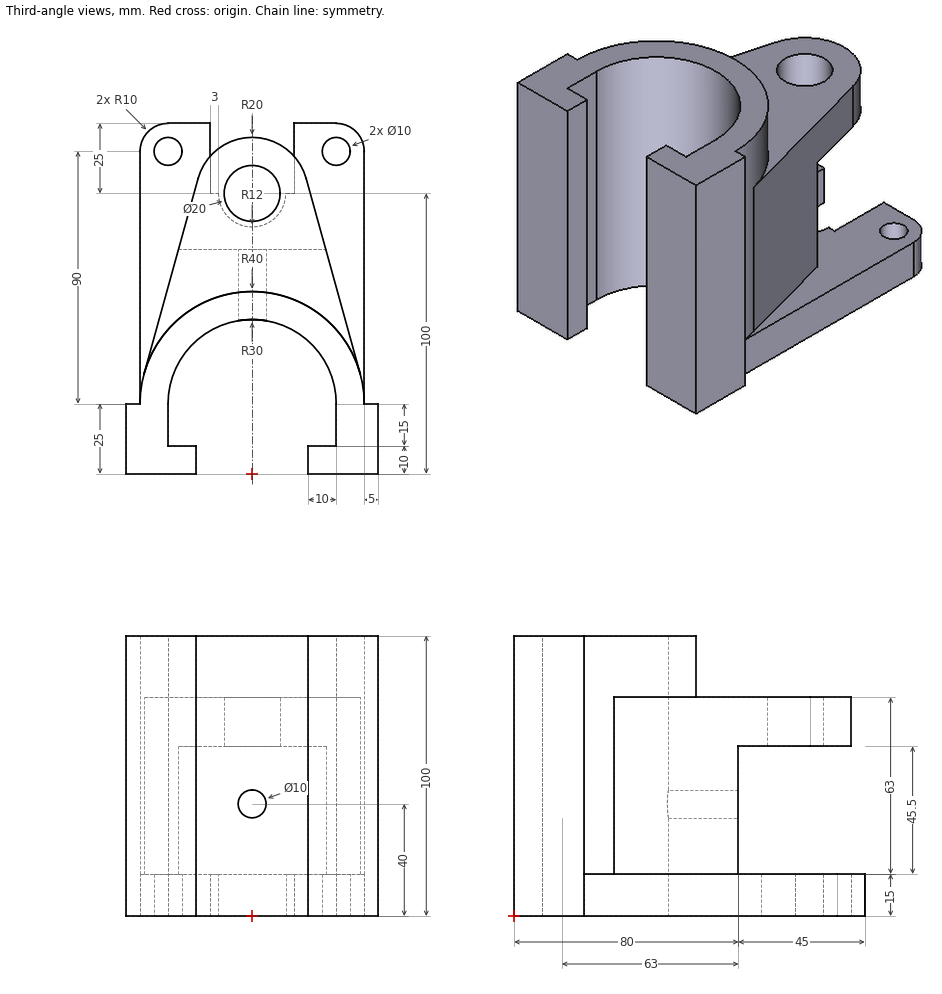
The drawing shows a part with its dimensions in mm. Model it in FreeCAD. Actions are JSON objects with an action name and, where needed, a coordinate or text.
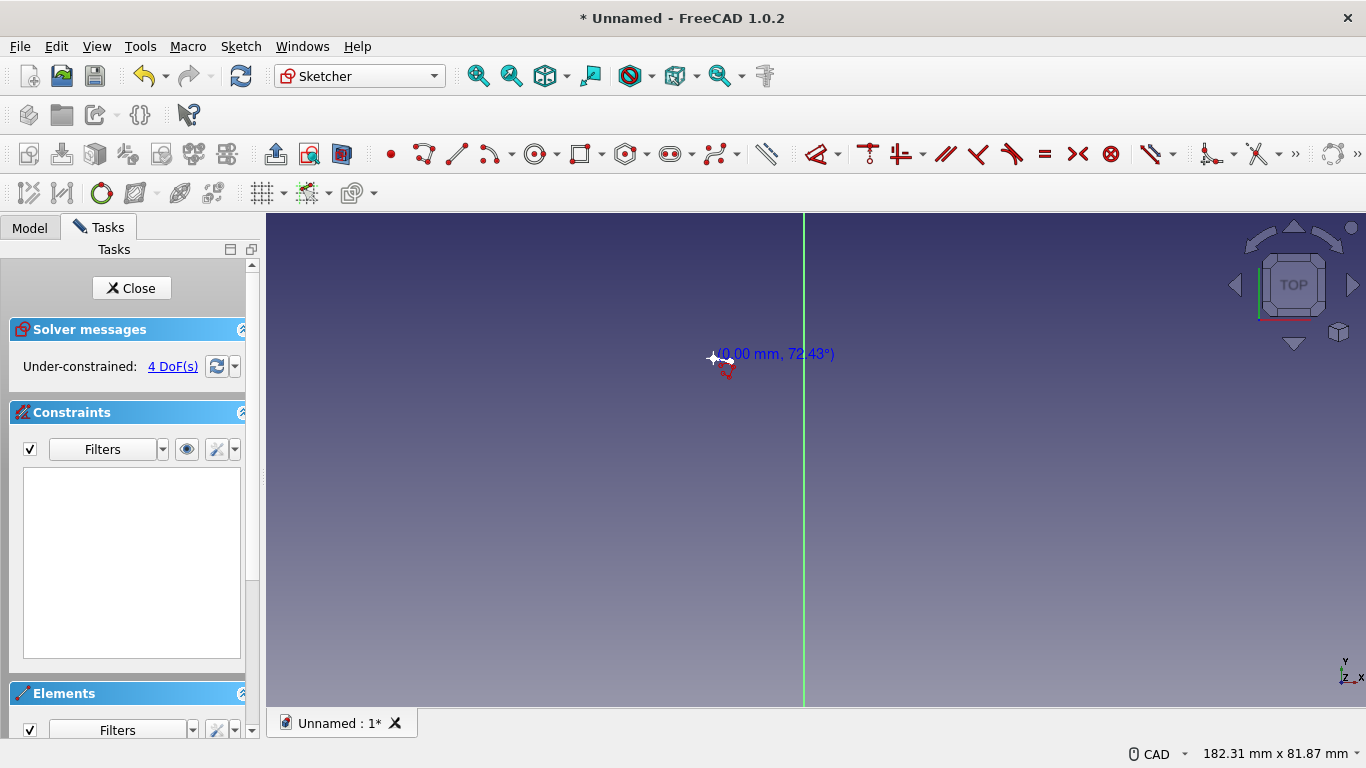
{"action": "scroll", "coordinate": [702, 358], "scroll_direction": "down", "scroll_amount": 4}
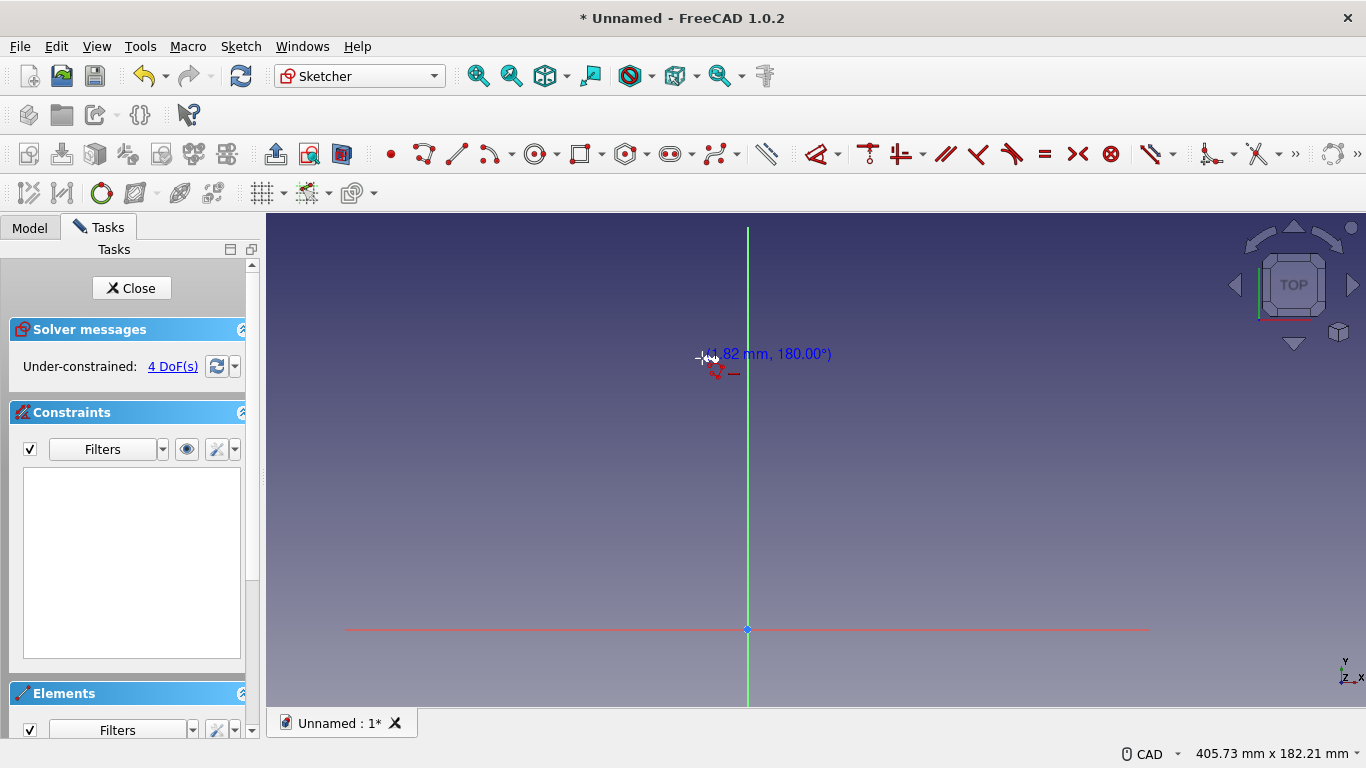
{"action": "left_click", "coordinate": [707, 291]}
{"action": "left_click", "coordinate": [667, 291]}
{"action": "right_click", "coordinate": [667, 291]}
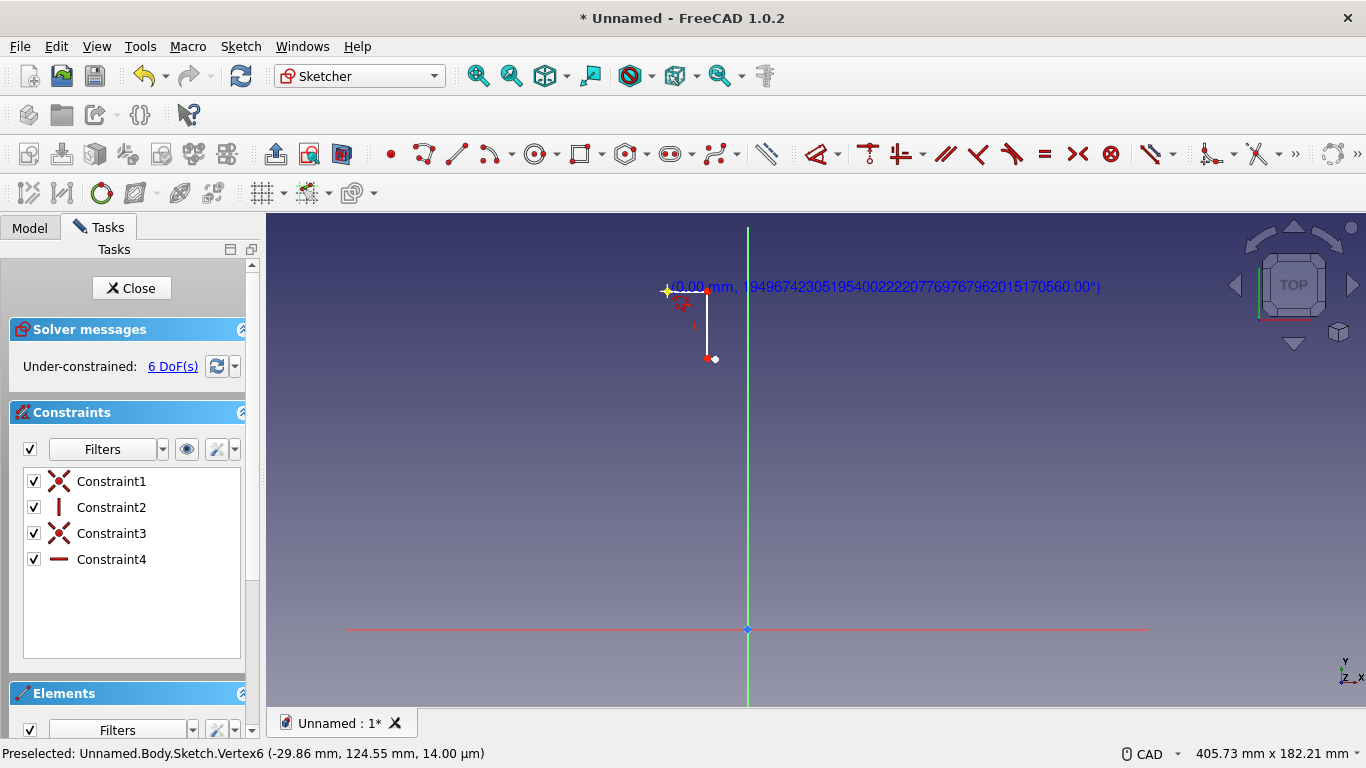
{"action": "key", "text": "g l"}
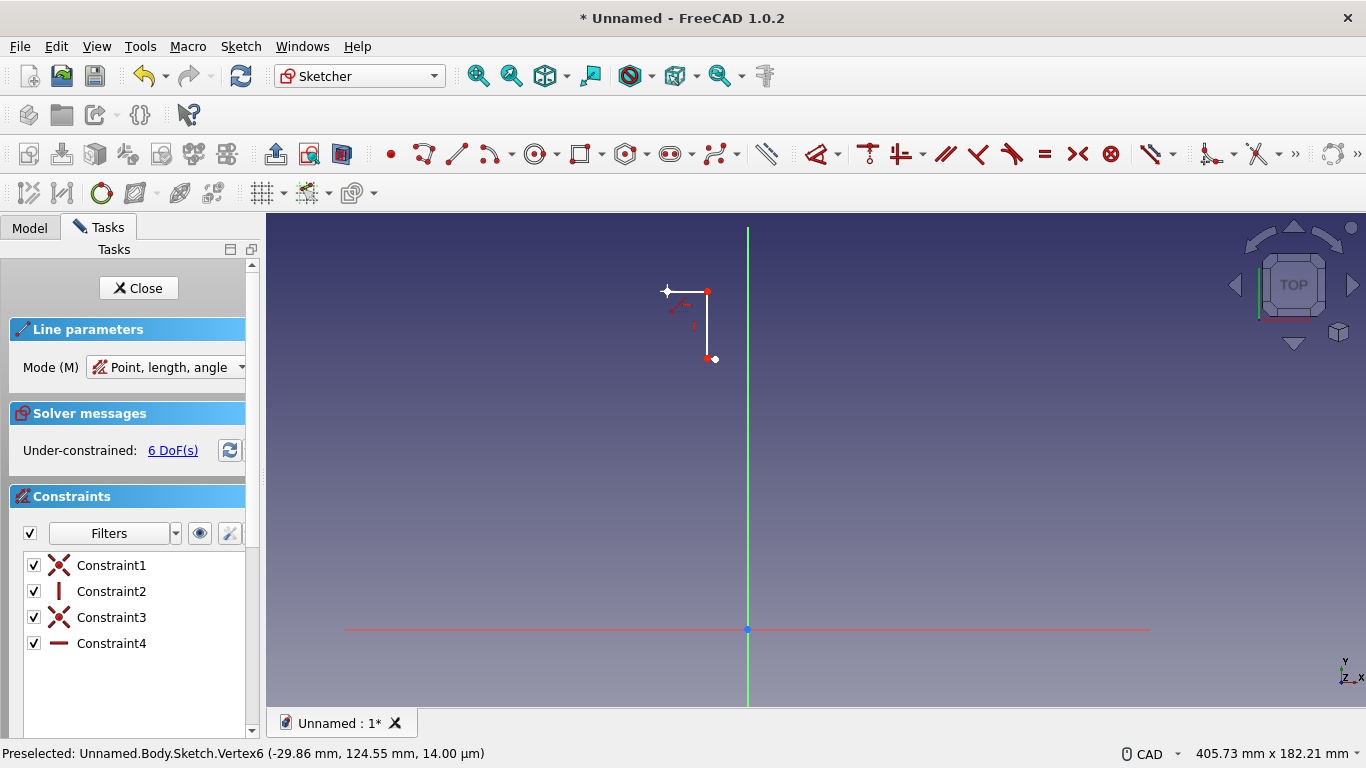
{"action": "left_click", "coordinate": [640, 318]}
{"action": "left_click", "coordinate": [640, 562]}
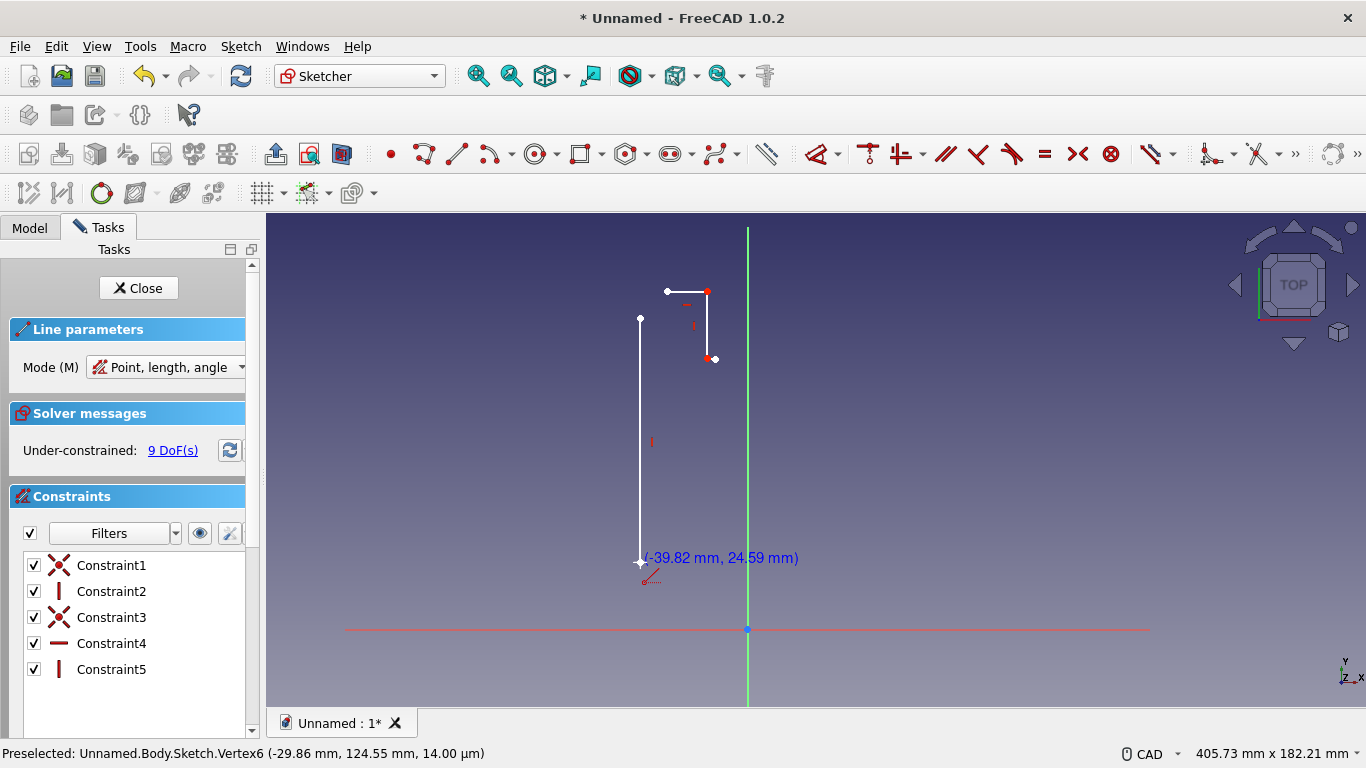
{"action": "left_click", "coordinate": [856, 562]}
{"action": "left_click", "coordinate": [856, 318]}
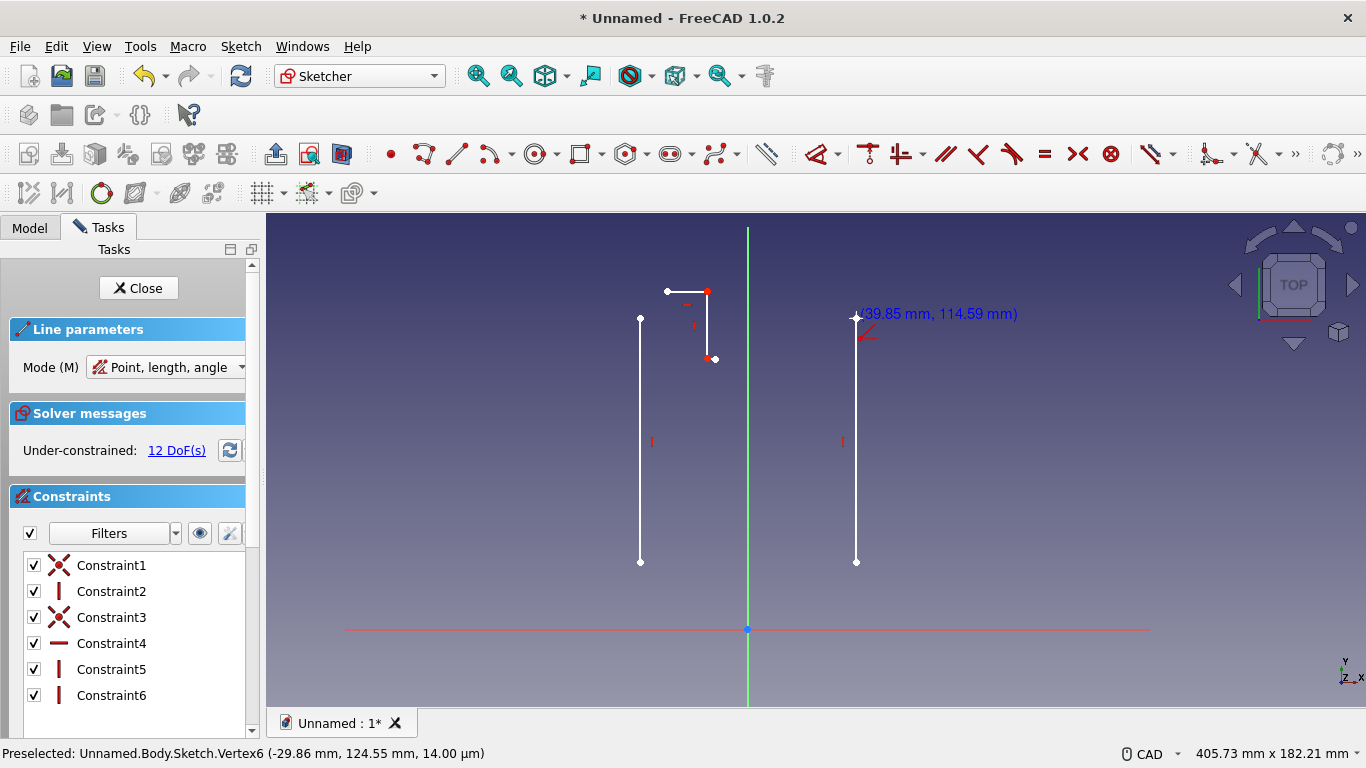
{"action": "left_click", "coordinate": [424, 154]}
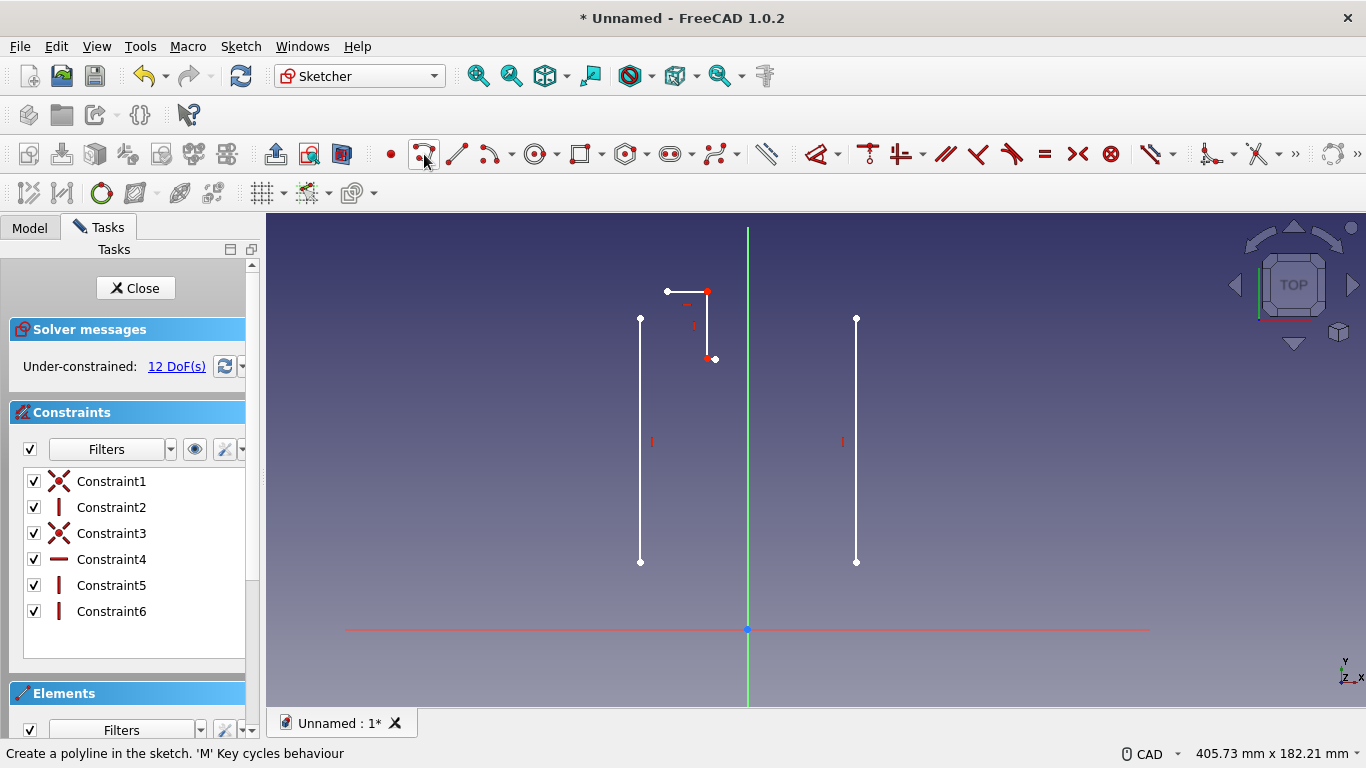
{"action": "left_click", "coordinate": [829, 291]}
{"action": "left_click", "coordinate": [789, 291]}
{"action": "left_click", "coordinate": [789, 359]}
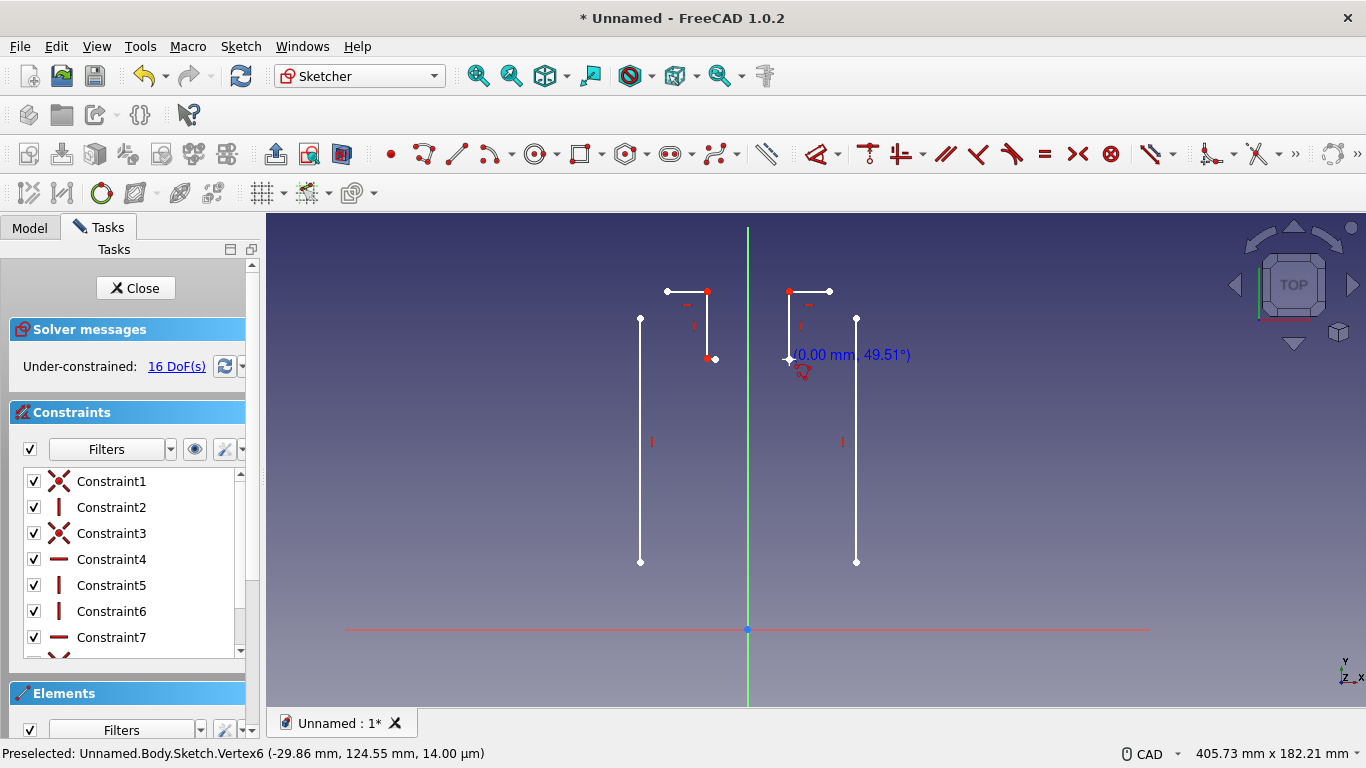
{"action": "scroll", "coordinate": [780, 359], "scroll_direction": "up", "scroll_amount": 4}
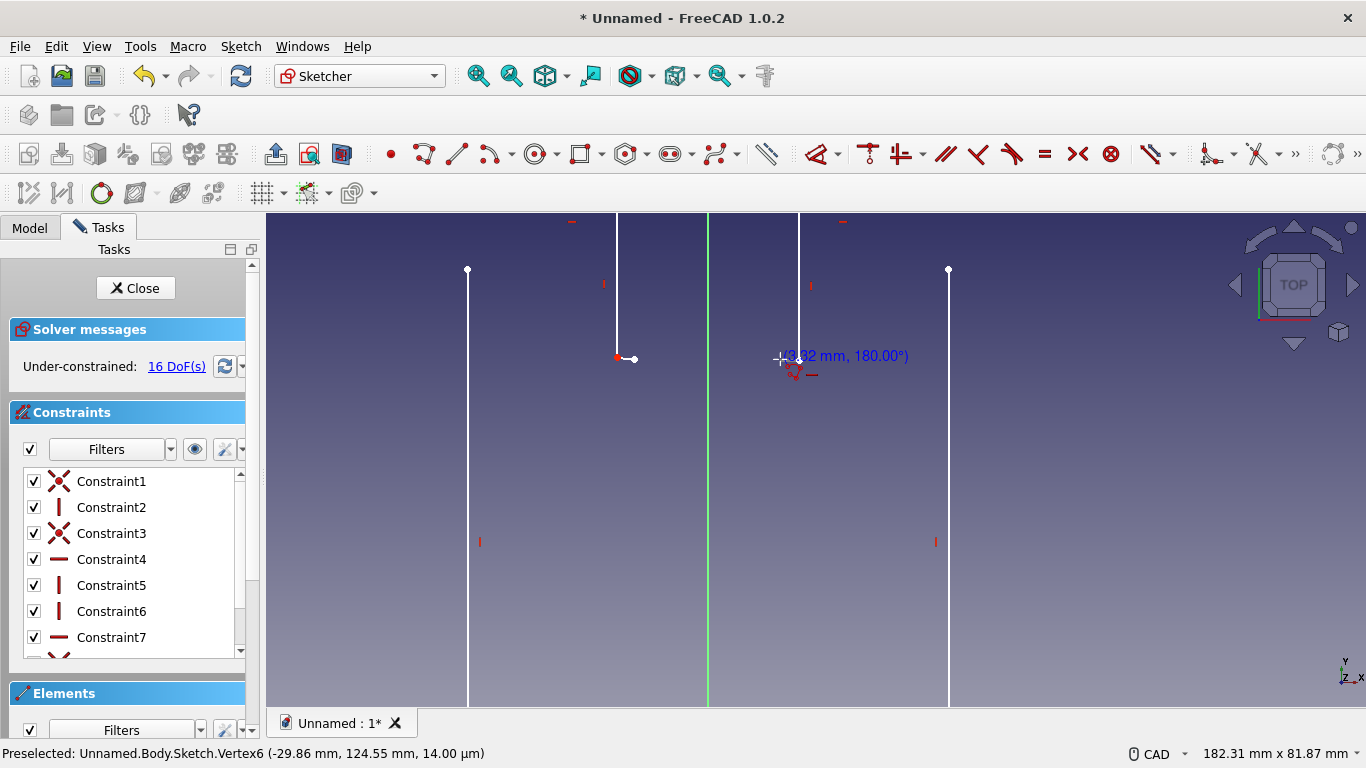
{"action": "left_click", "coordinate": [781, 359]}
{"action": "right_click", "coordinate": [781, 359]}